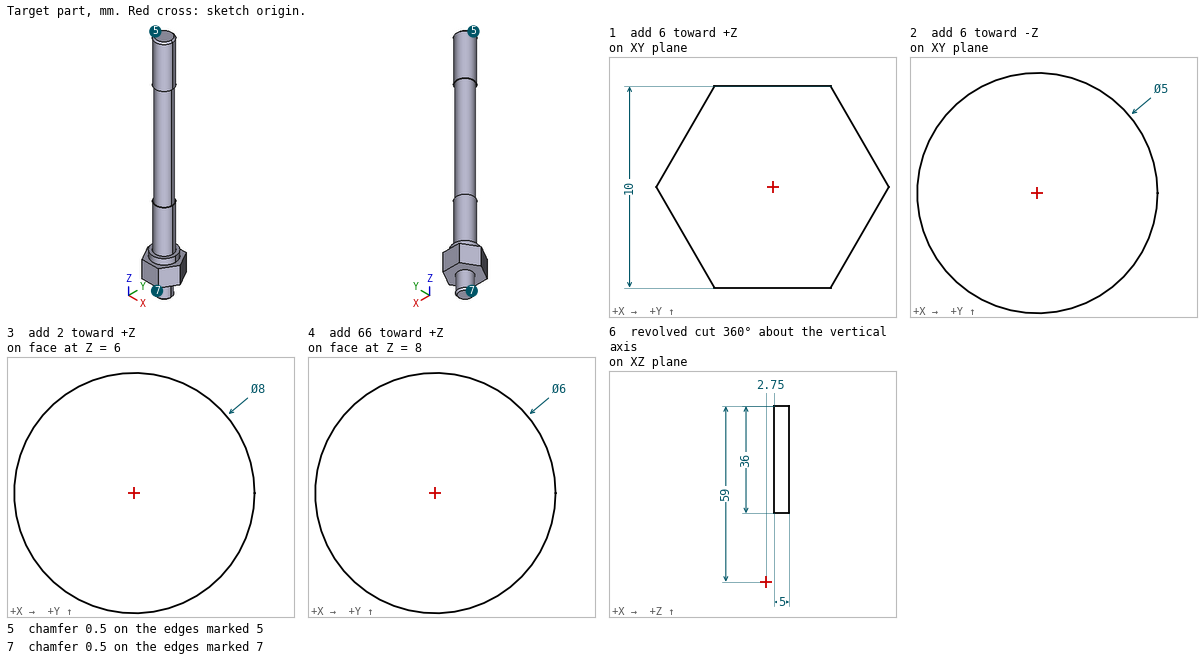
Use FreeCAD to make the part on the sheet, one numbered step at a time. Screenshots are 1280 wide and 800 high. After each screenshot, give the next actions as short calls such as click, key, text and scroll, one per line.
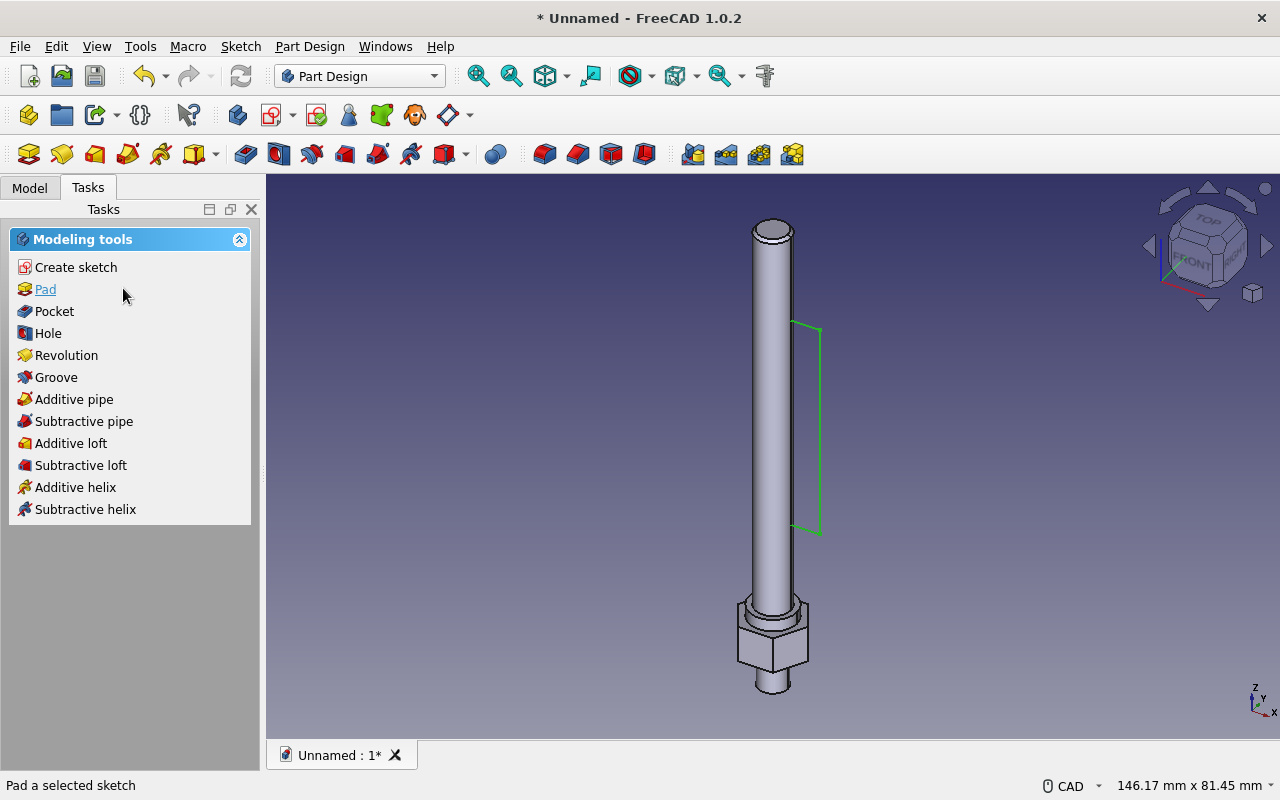
click(312, 154)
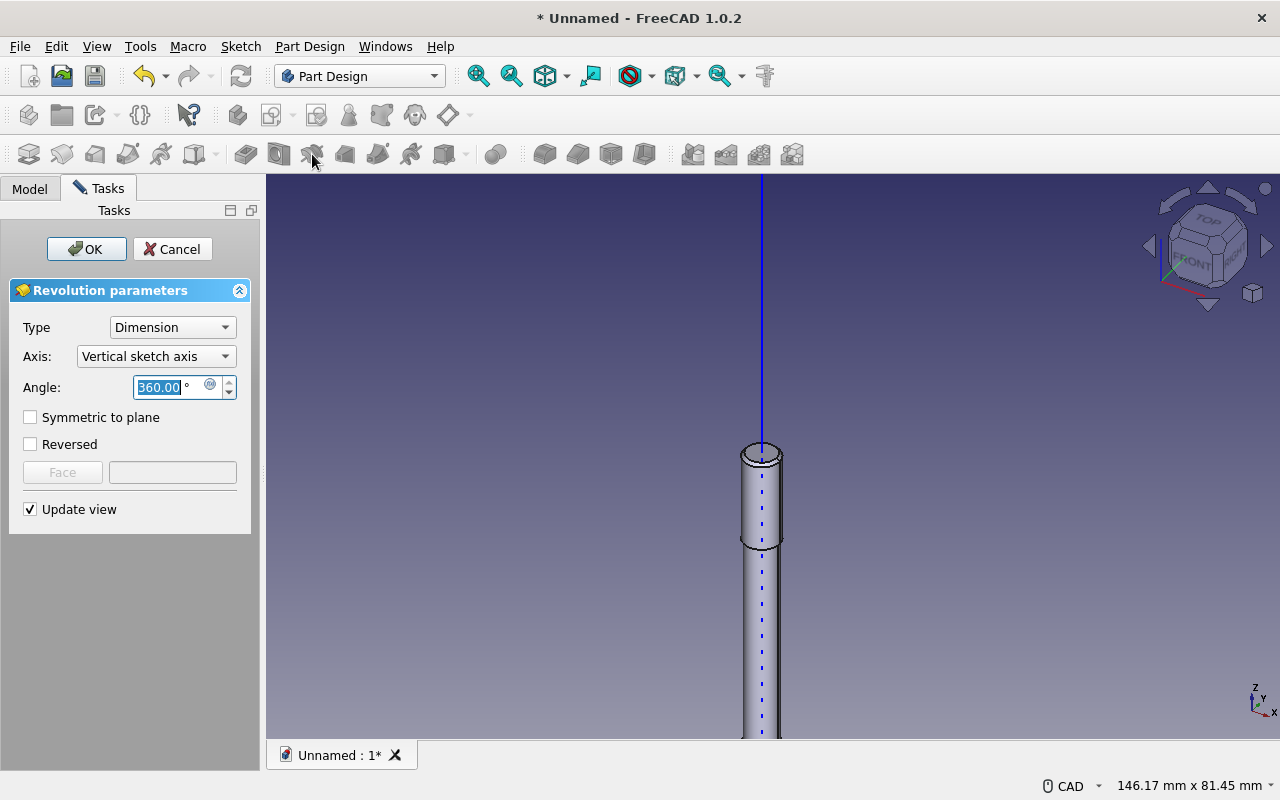
click(87, 249)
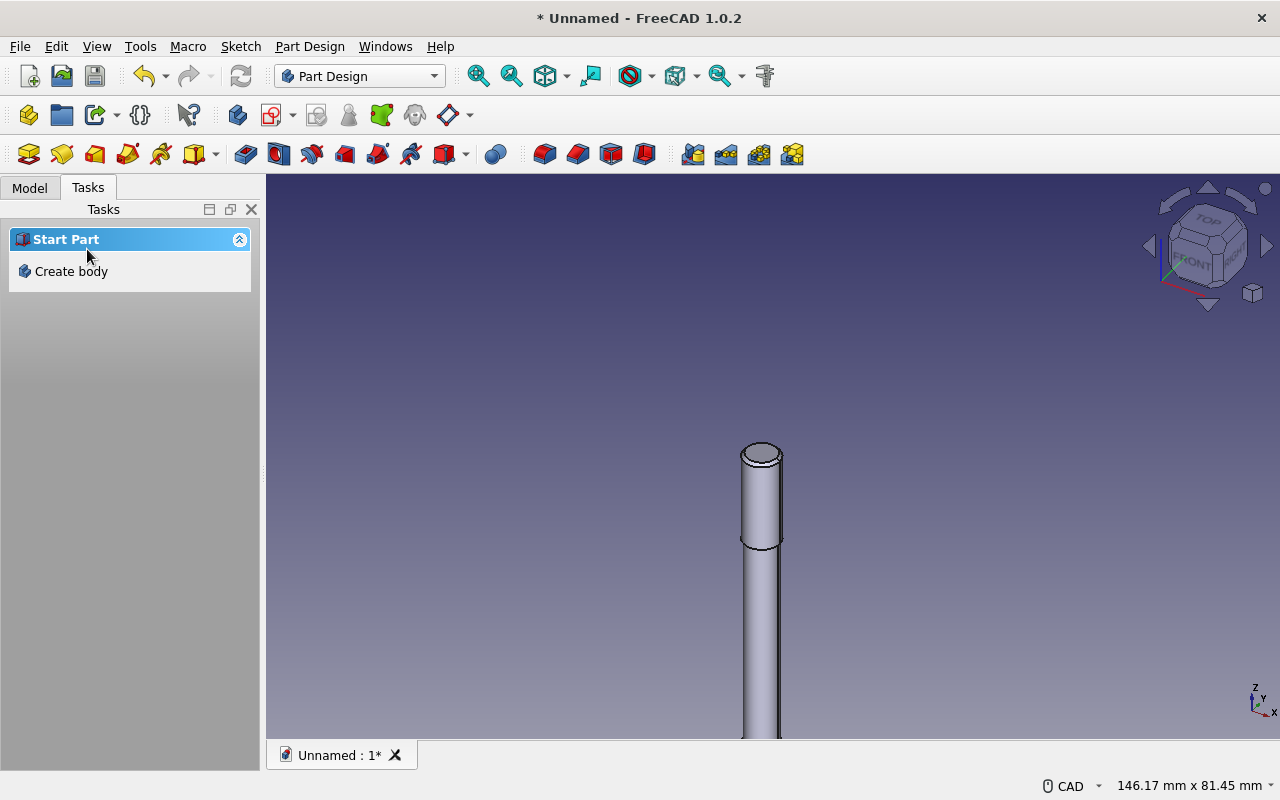
click(479, 76)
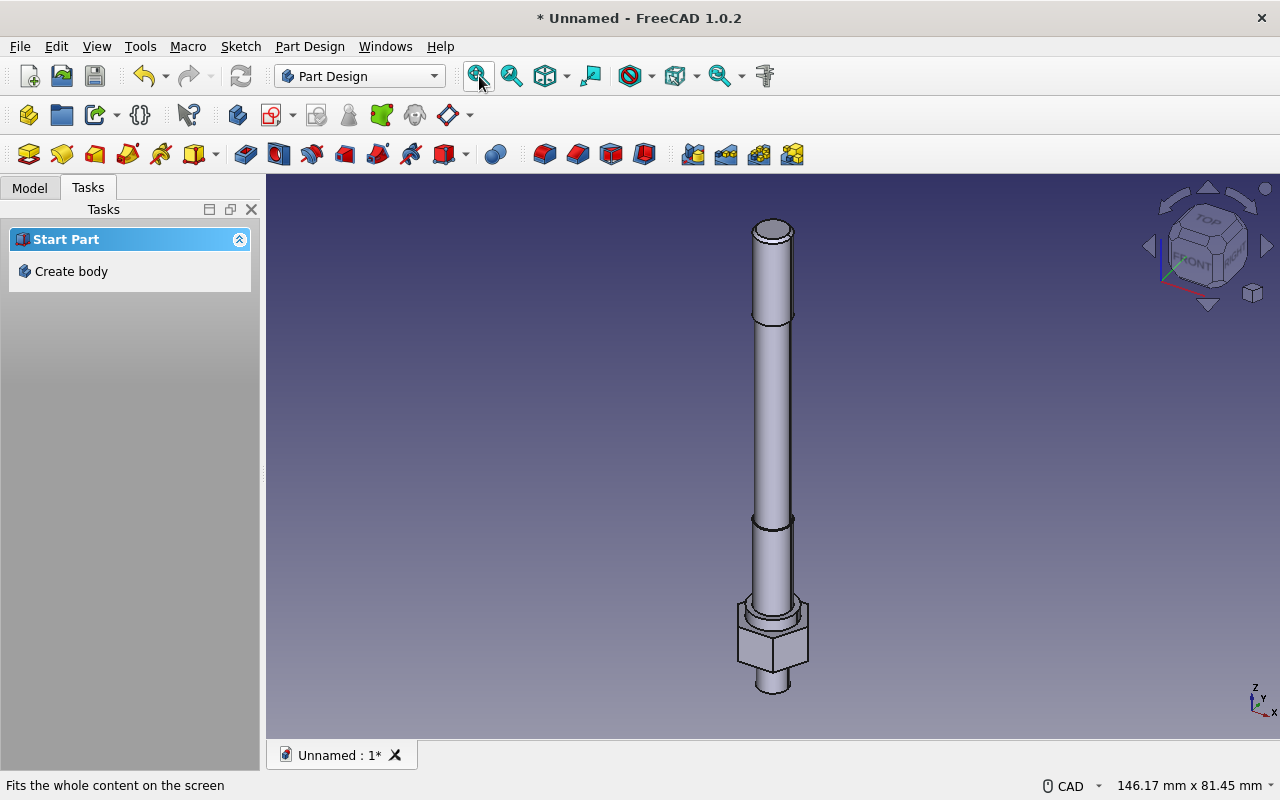
key(0)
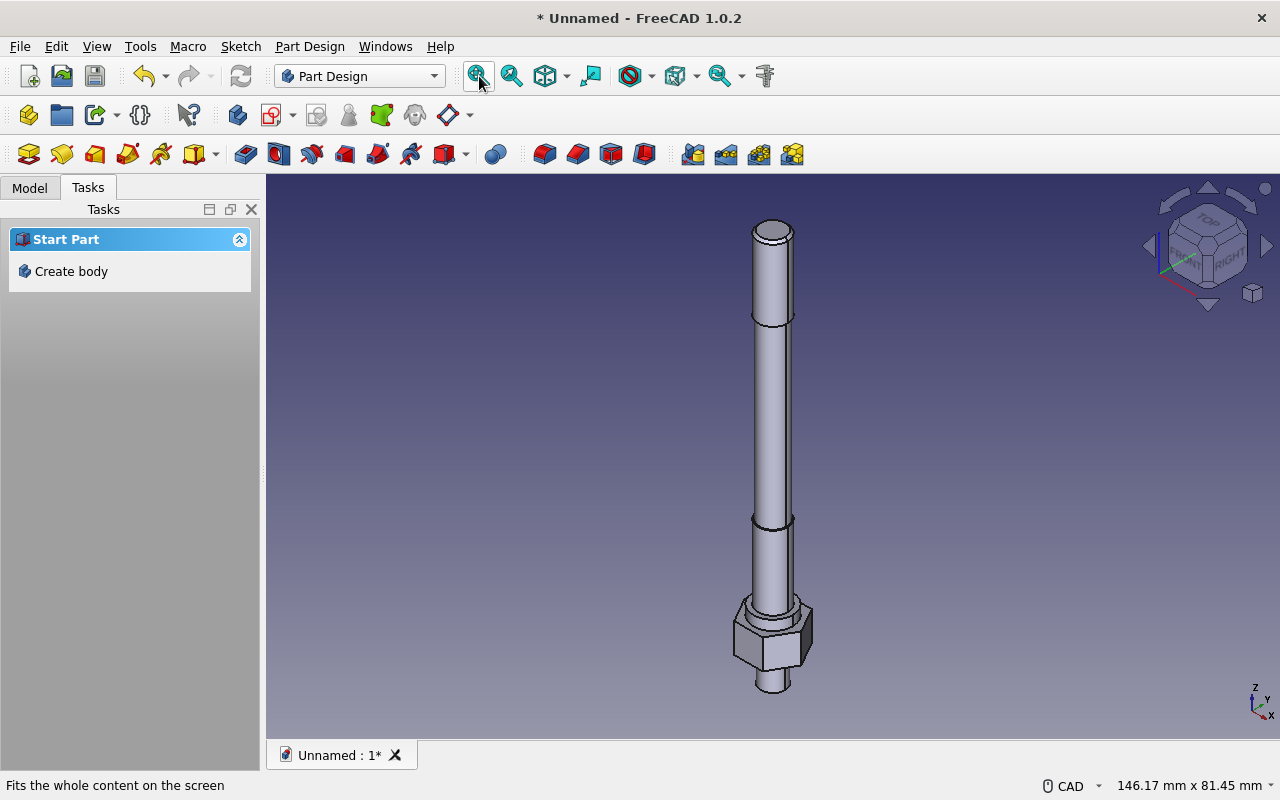
click(765, 691)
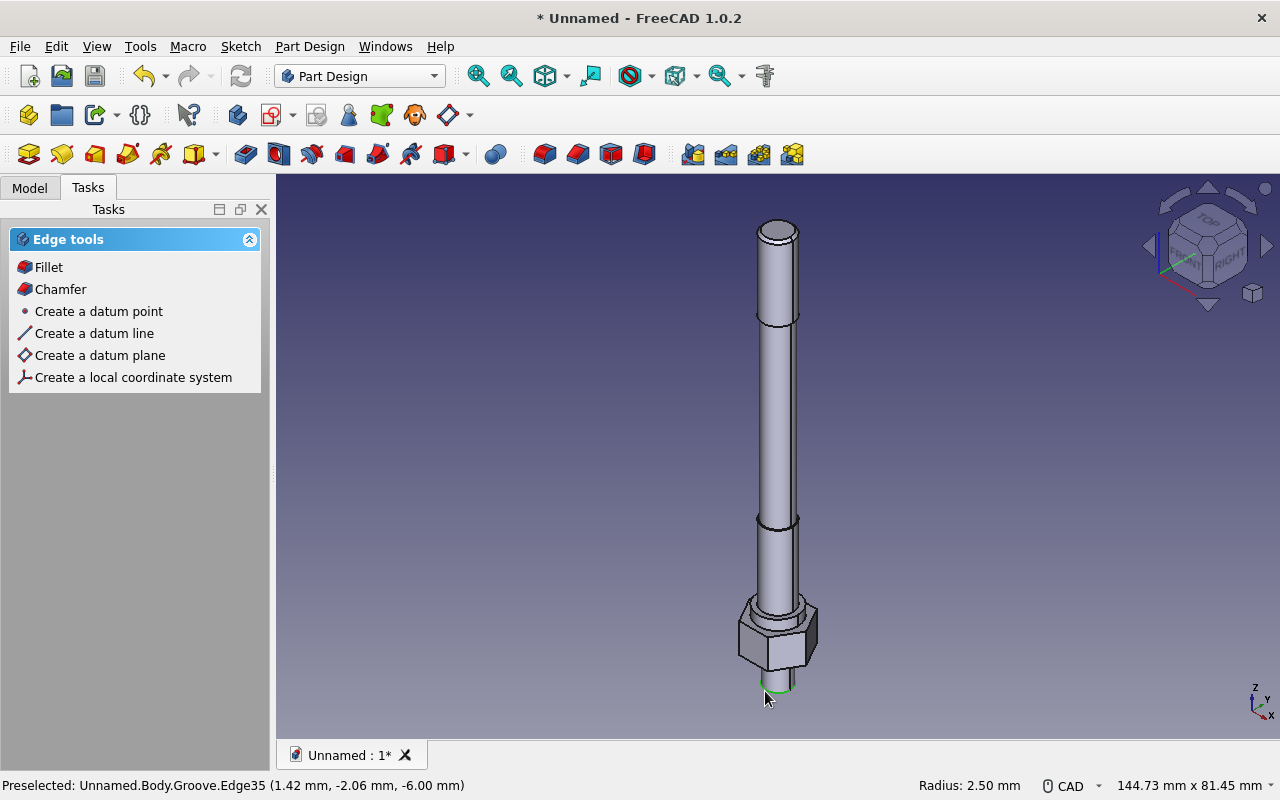
click(578, 154)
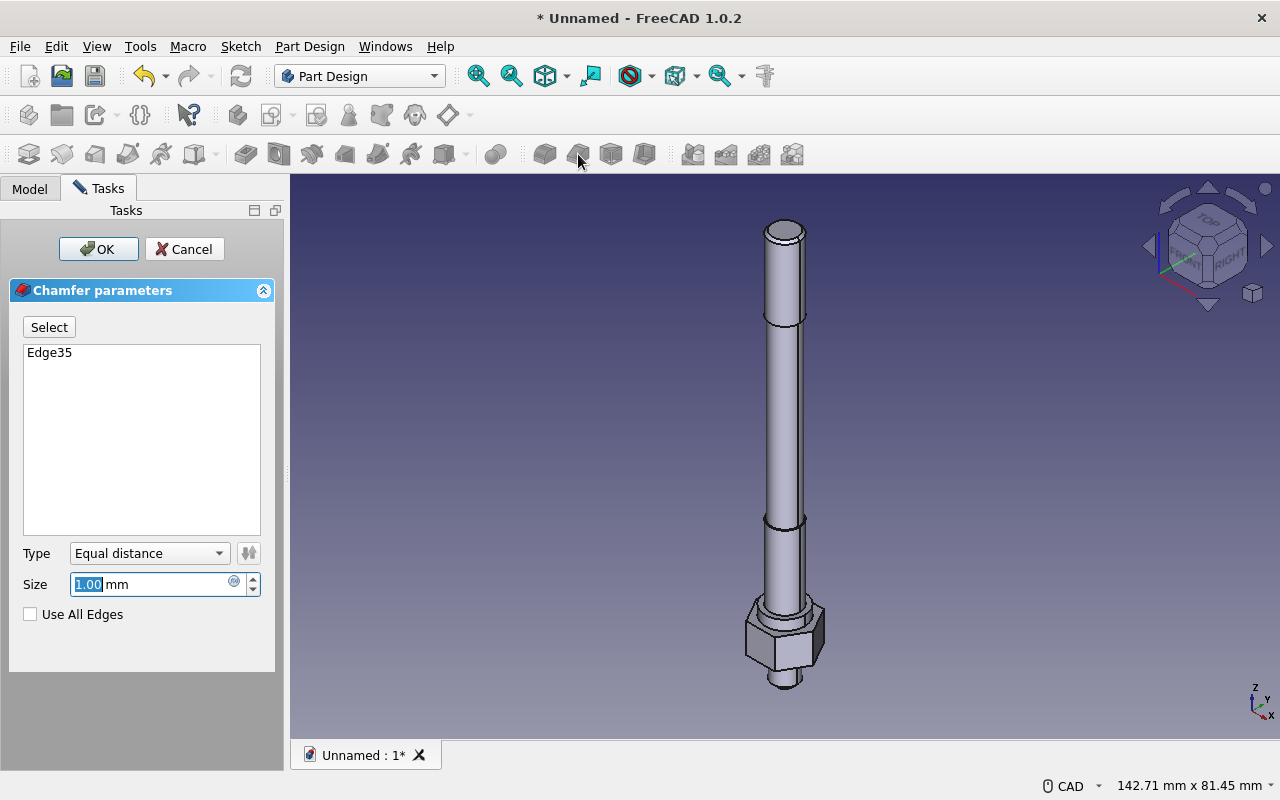
text(0.5)
key(Tab)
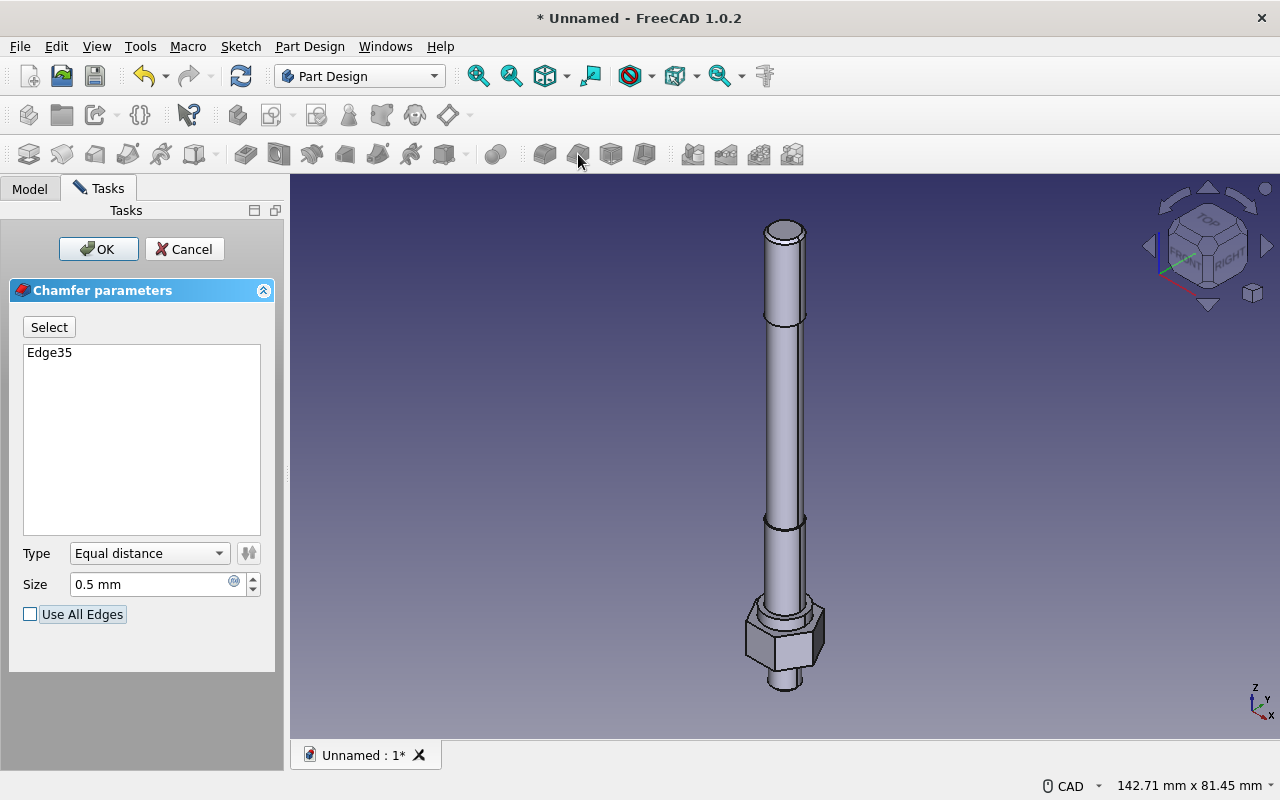
click(99, 249)